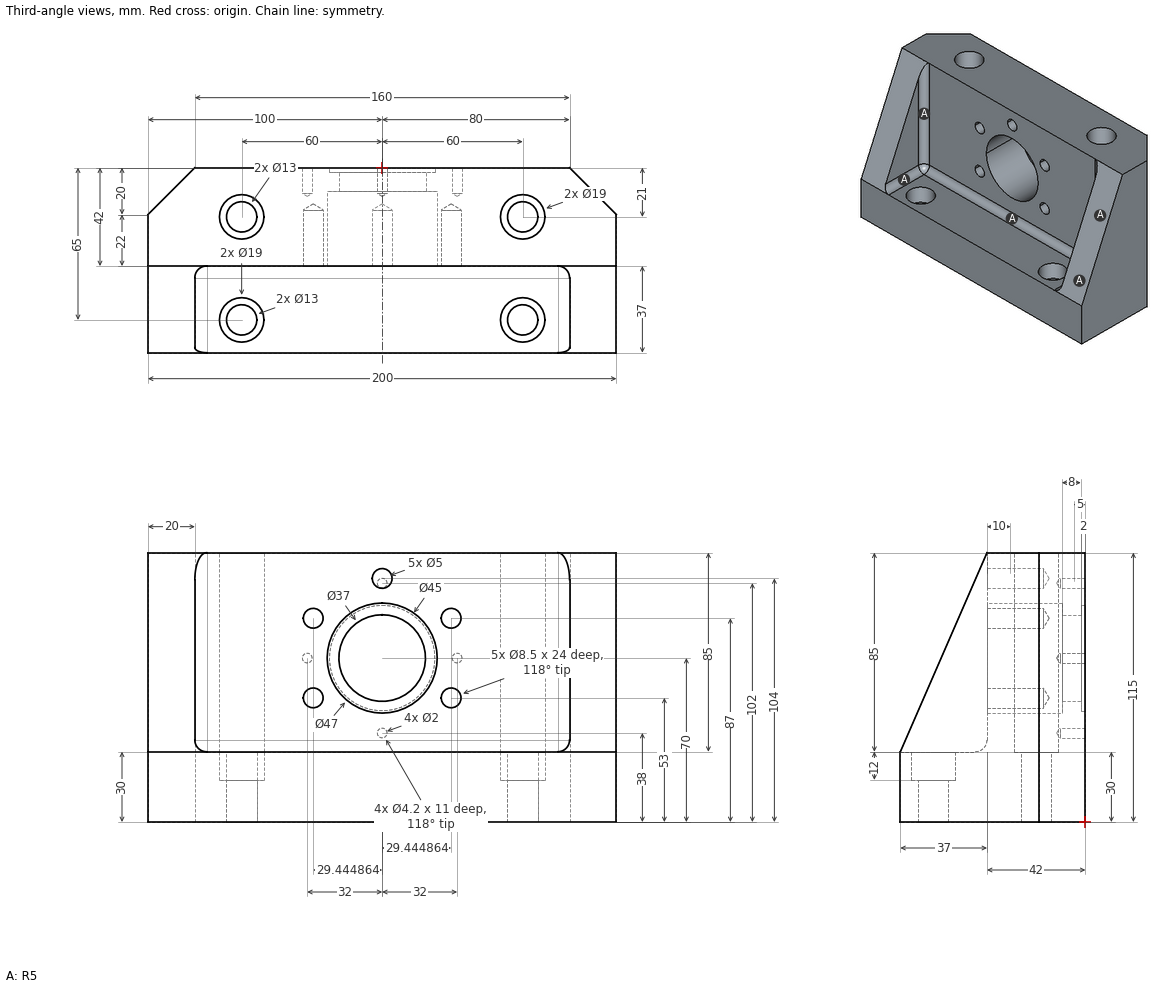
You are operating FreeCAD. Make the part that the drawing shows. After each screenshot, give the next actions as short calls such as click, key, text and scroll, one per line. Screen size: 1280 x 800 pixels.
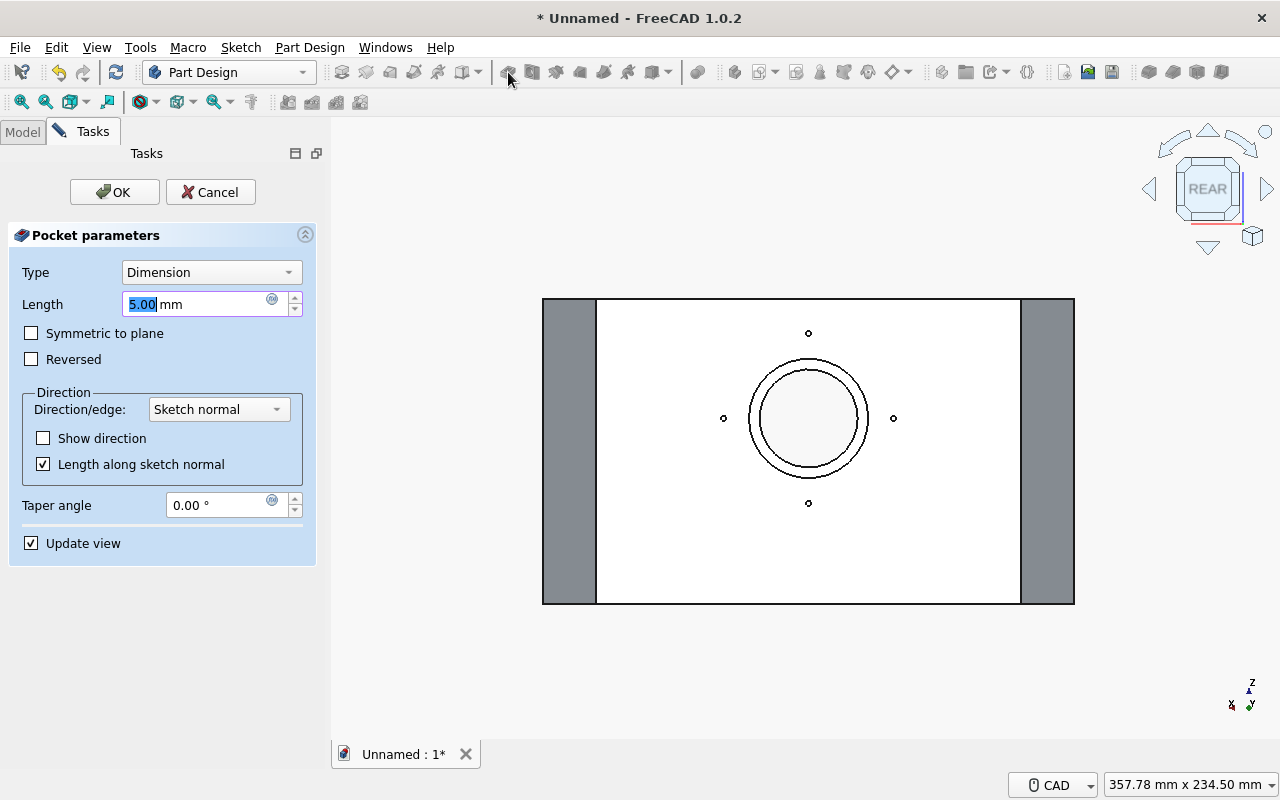
text(5)
key(Tab)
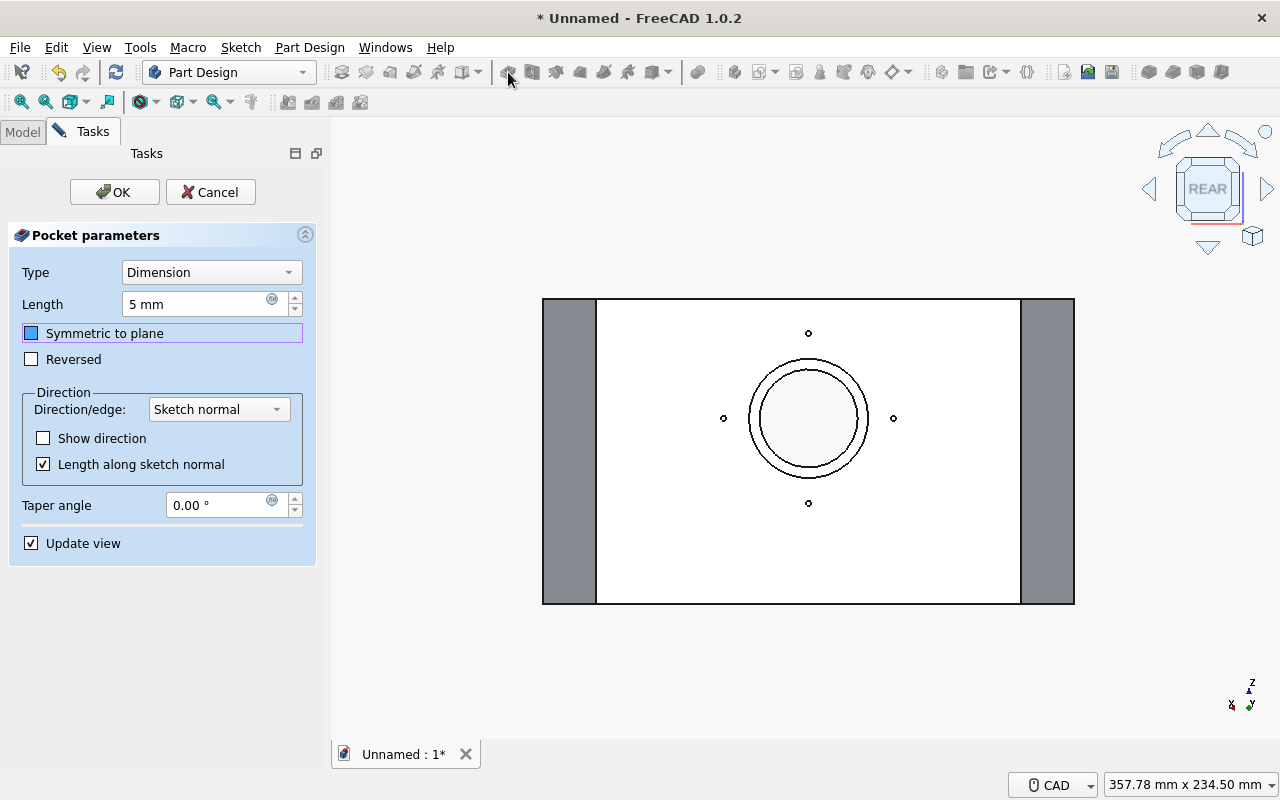
click(115, 192)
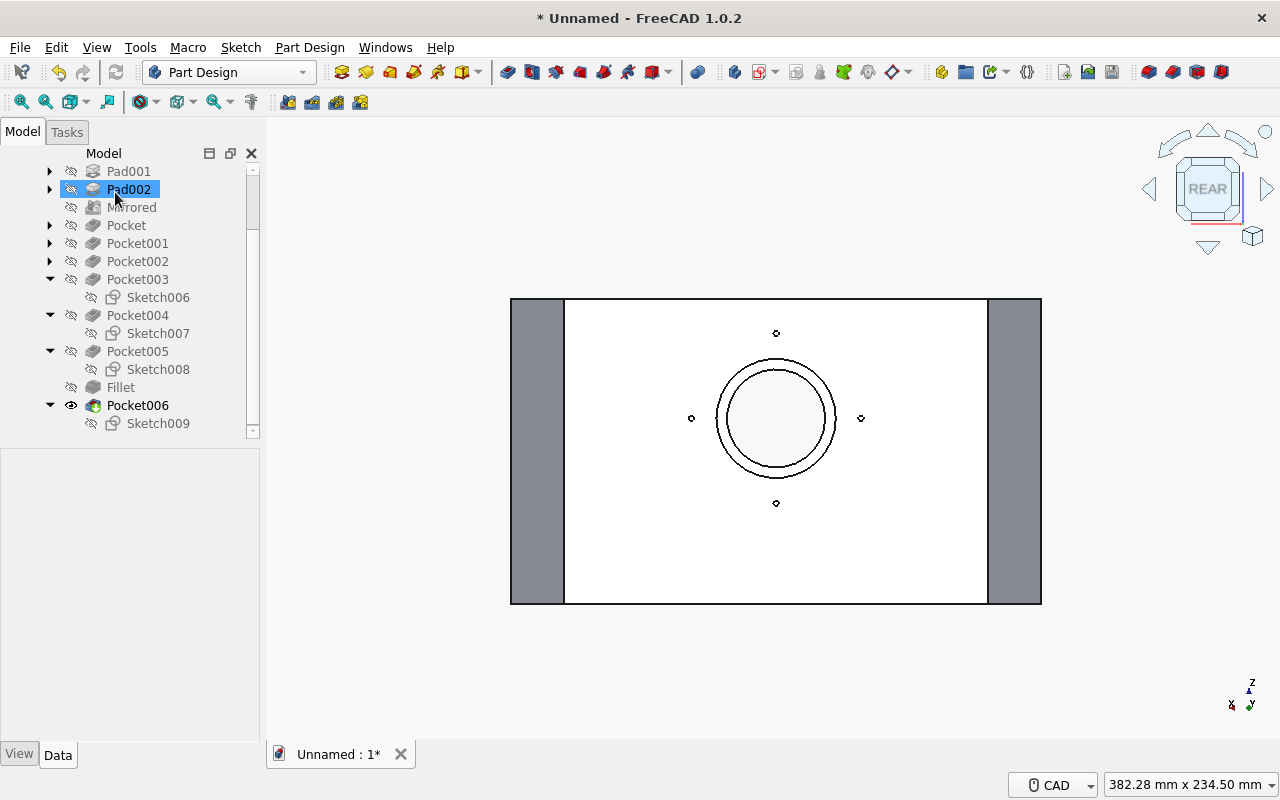
click(655, 494)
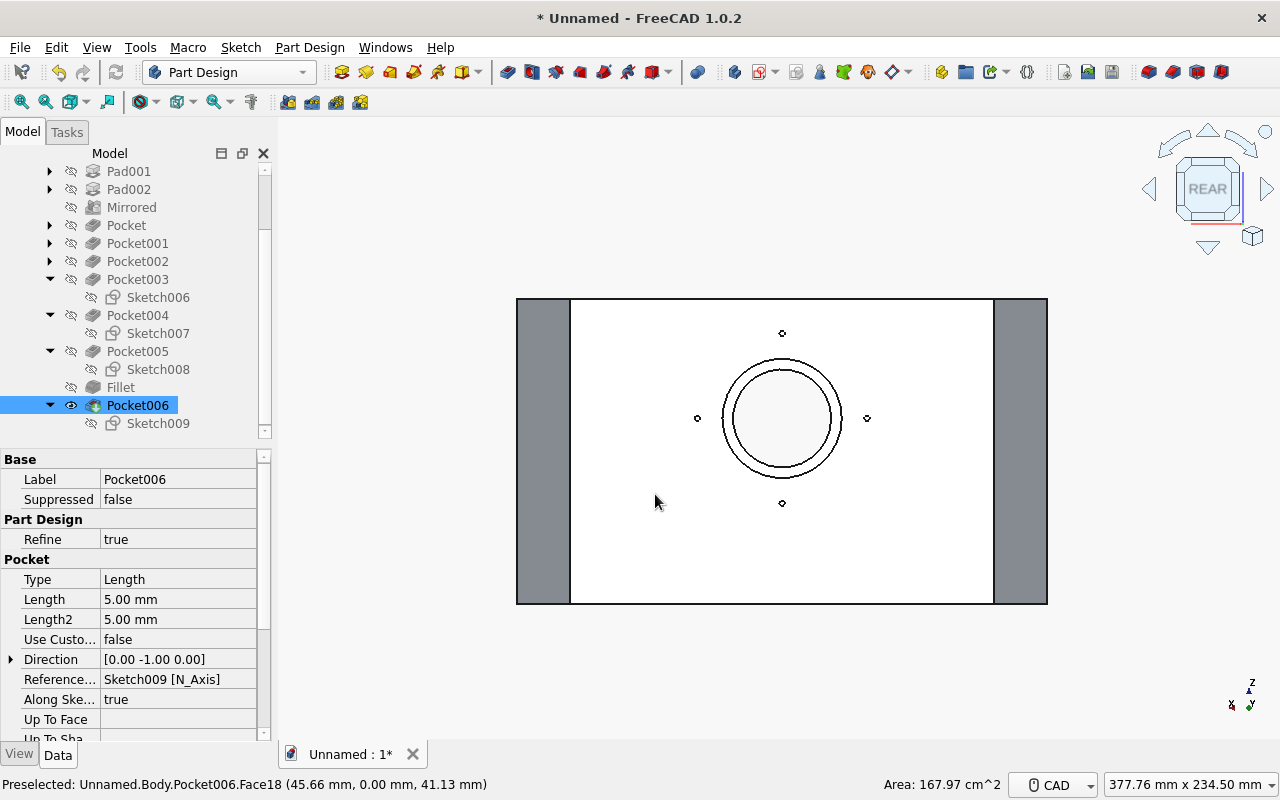
click(760, 72)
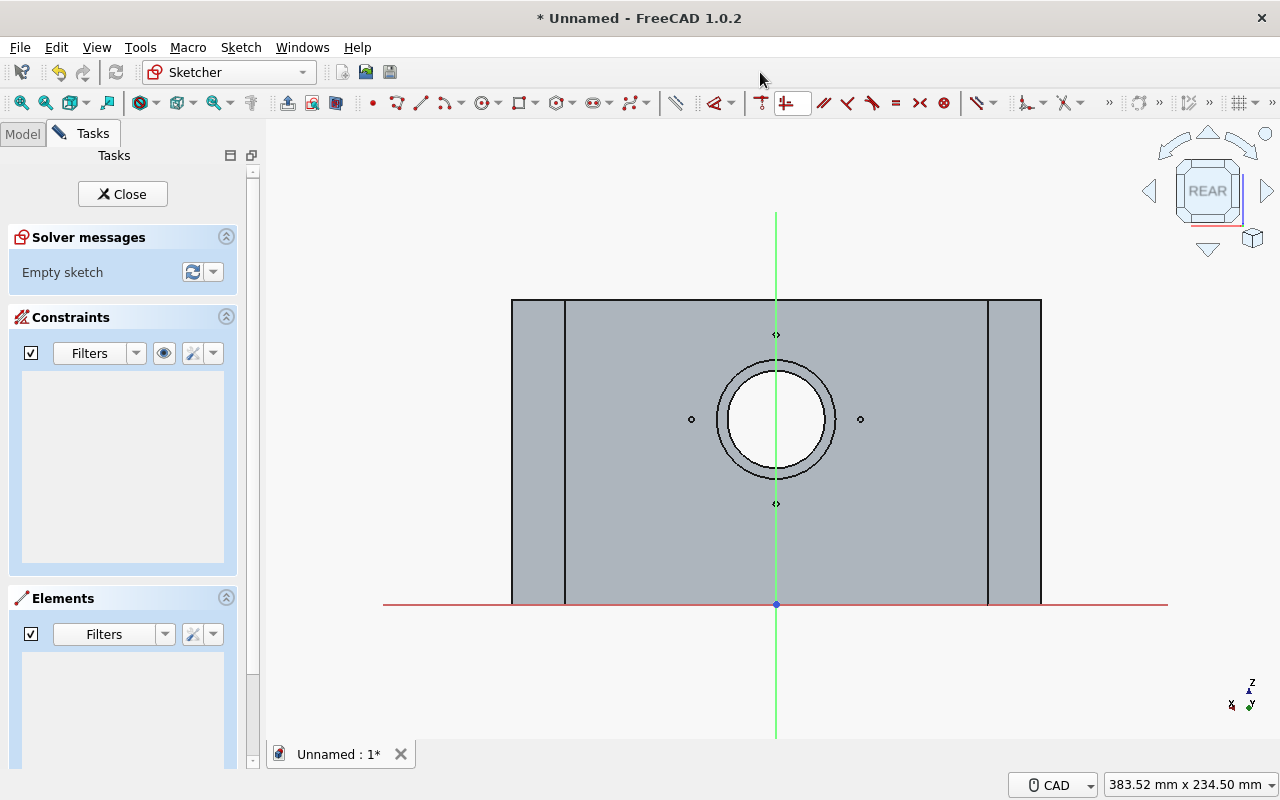
scroll(922, 544, up, 2)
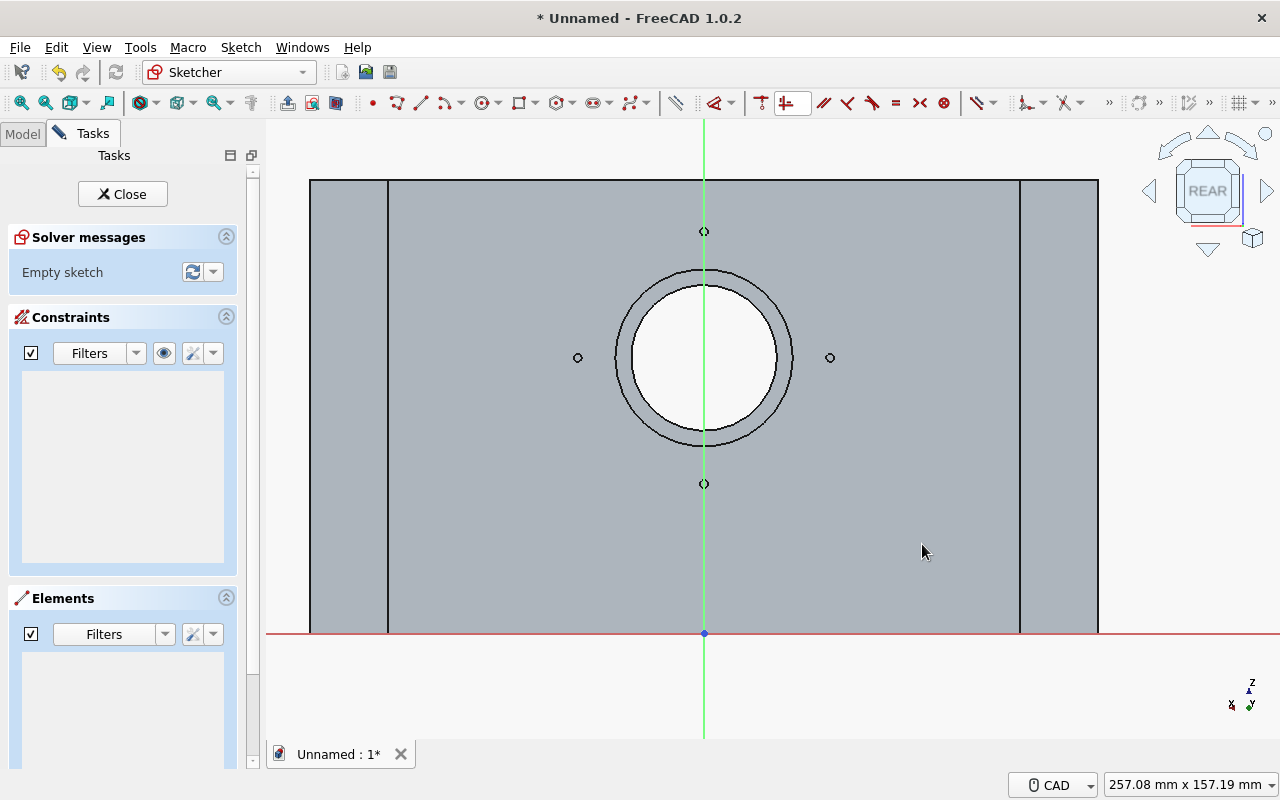
click(482, 104)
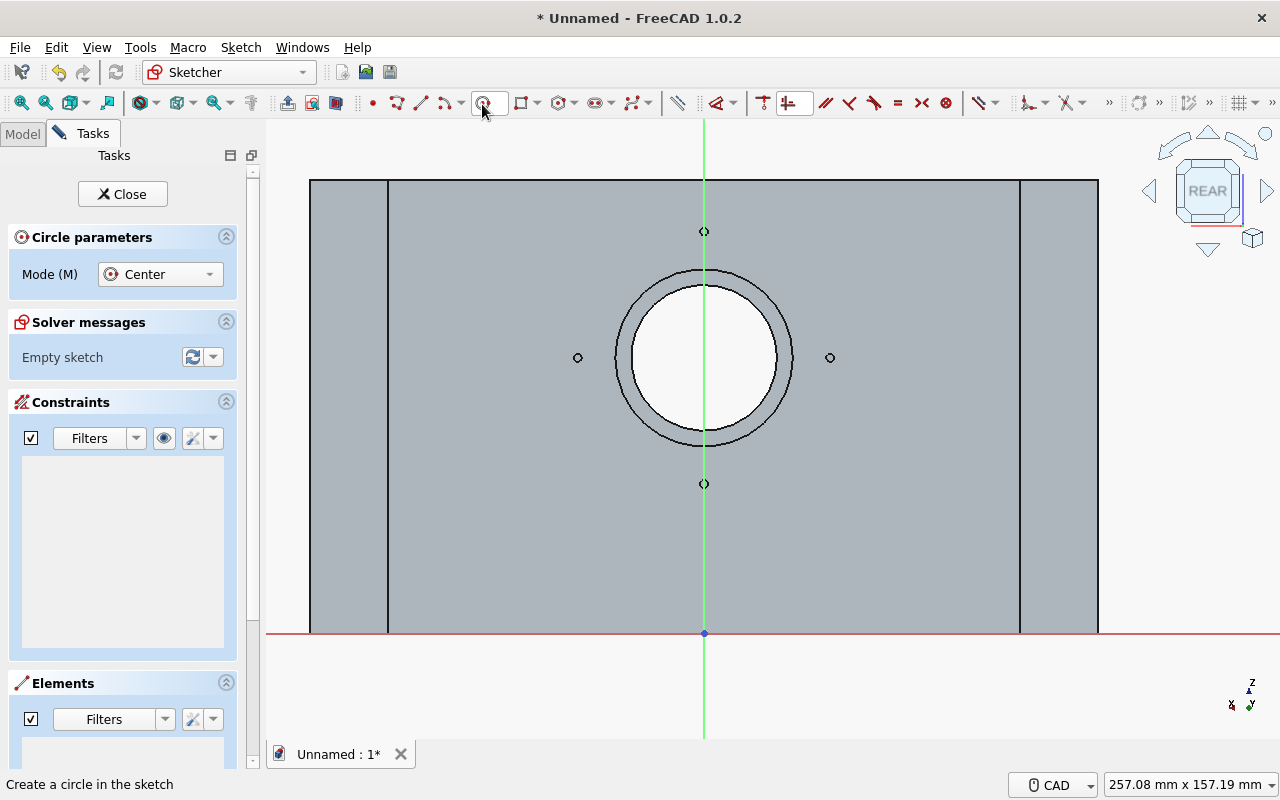
scroll(704, 484, up, 6)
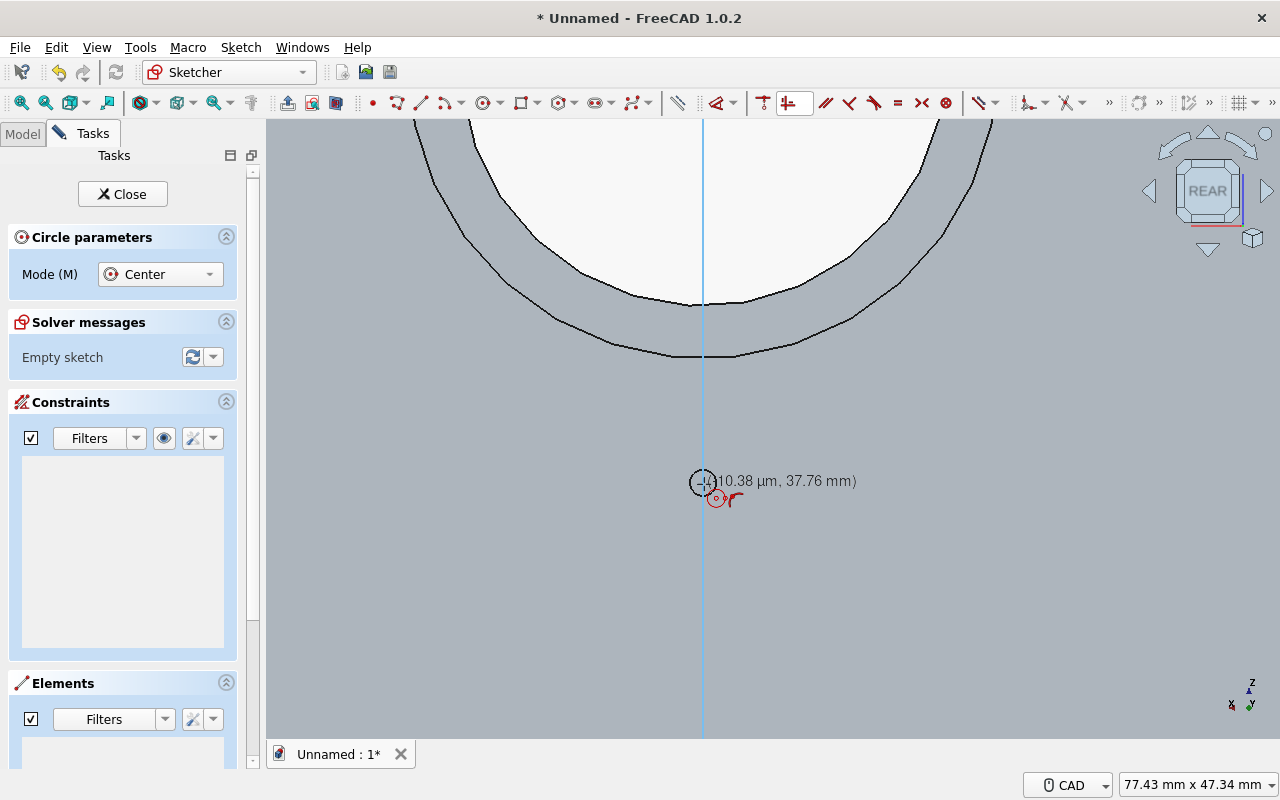
click(703, 483)
move(723, 463)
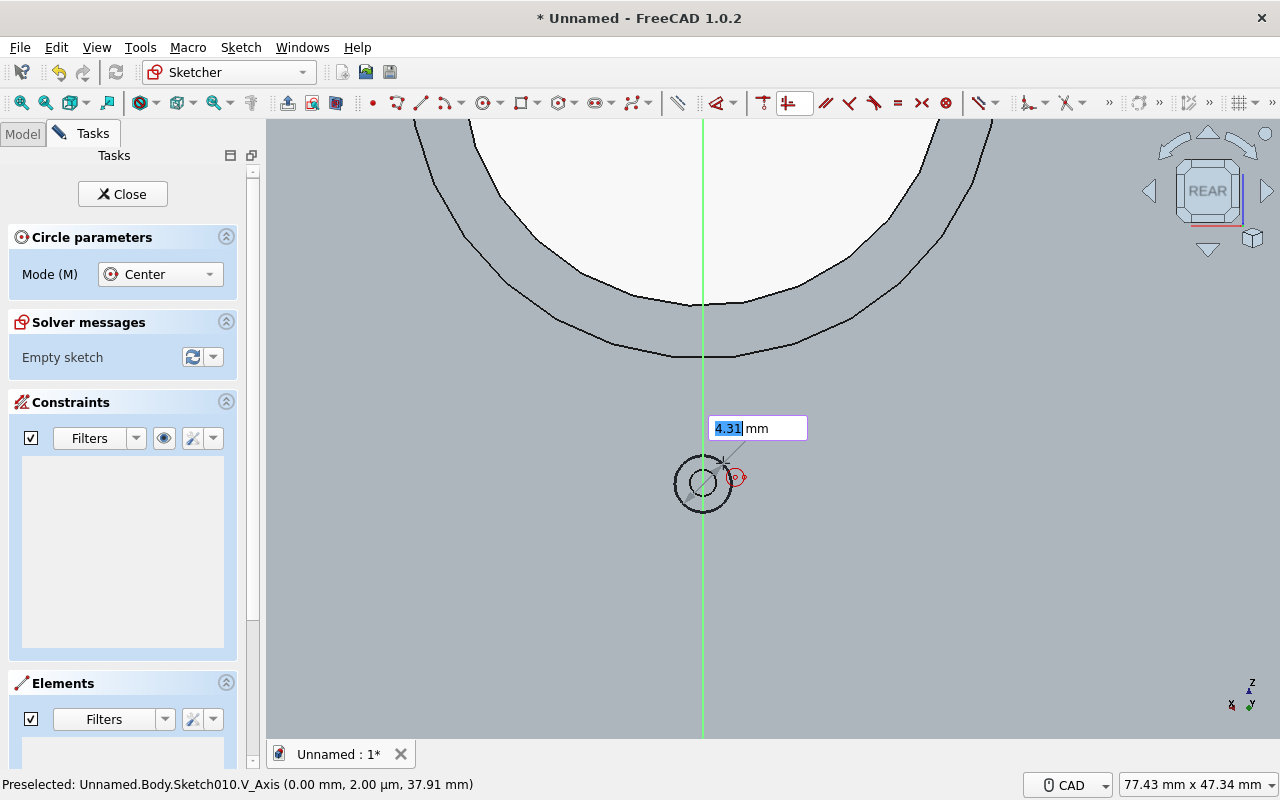
text(4.2)
key(Return)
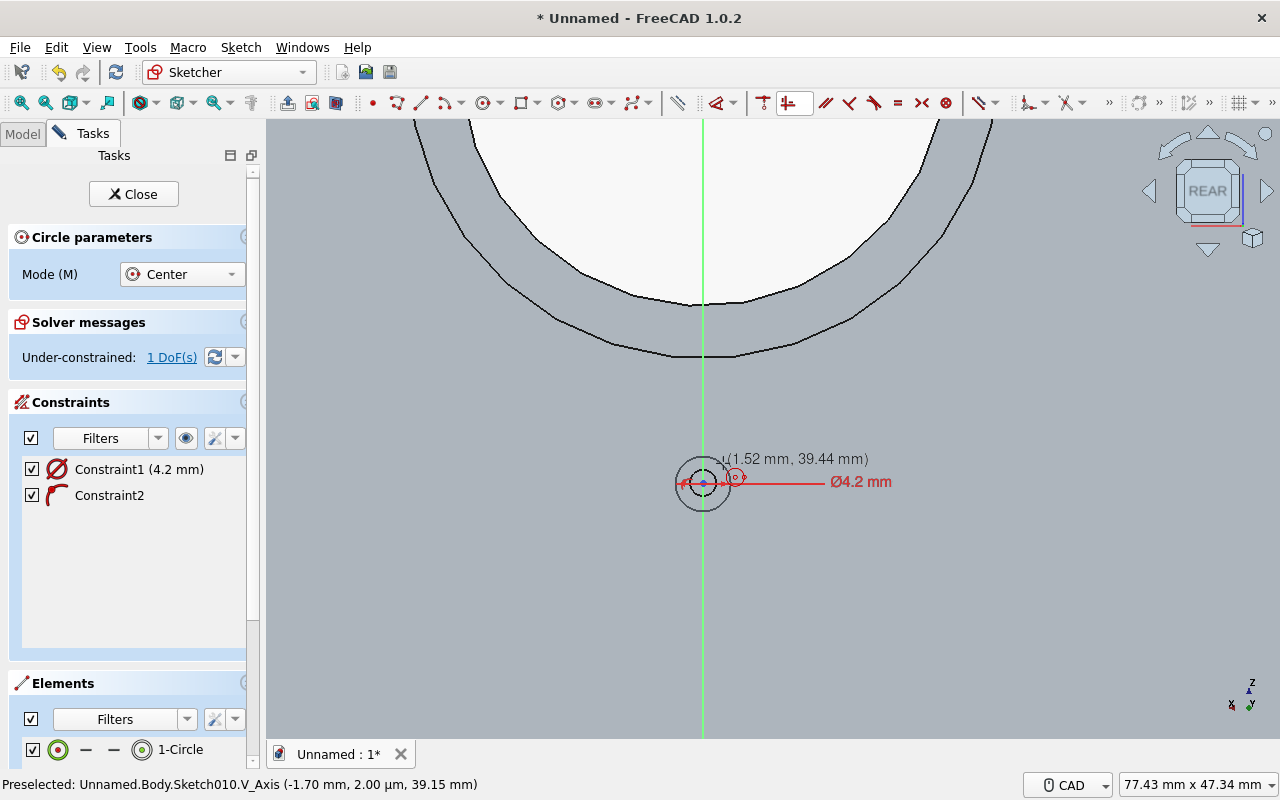
scroll(705, 485, down, 6)